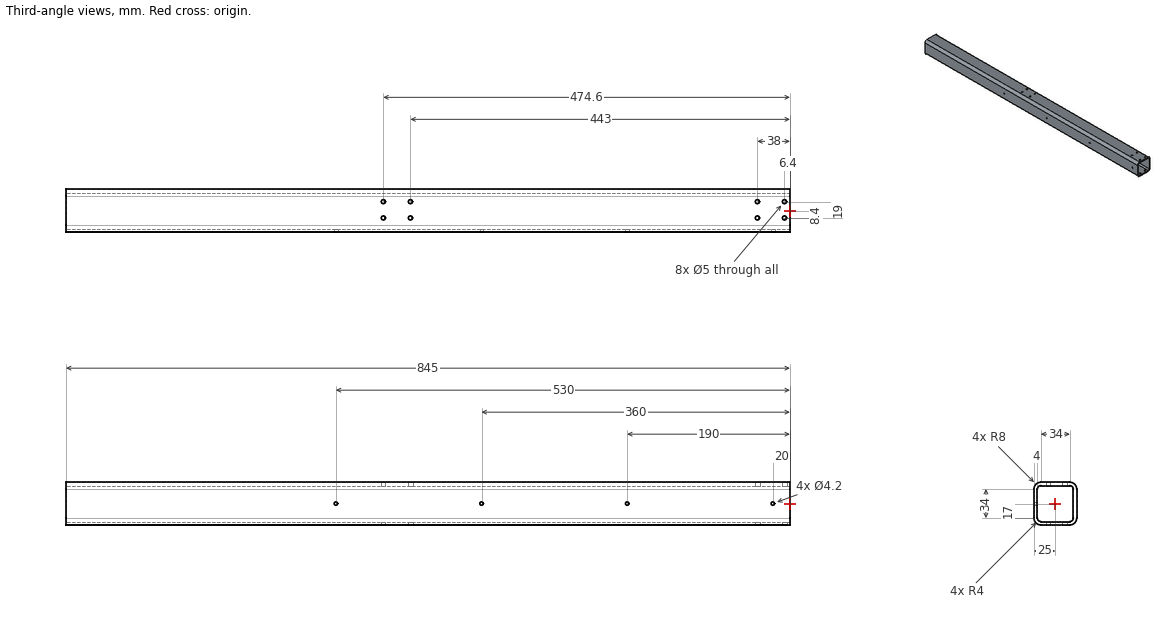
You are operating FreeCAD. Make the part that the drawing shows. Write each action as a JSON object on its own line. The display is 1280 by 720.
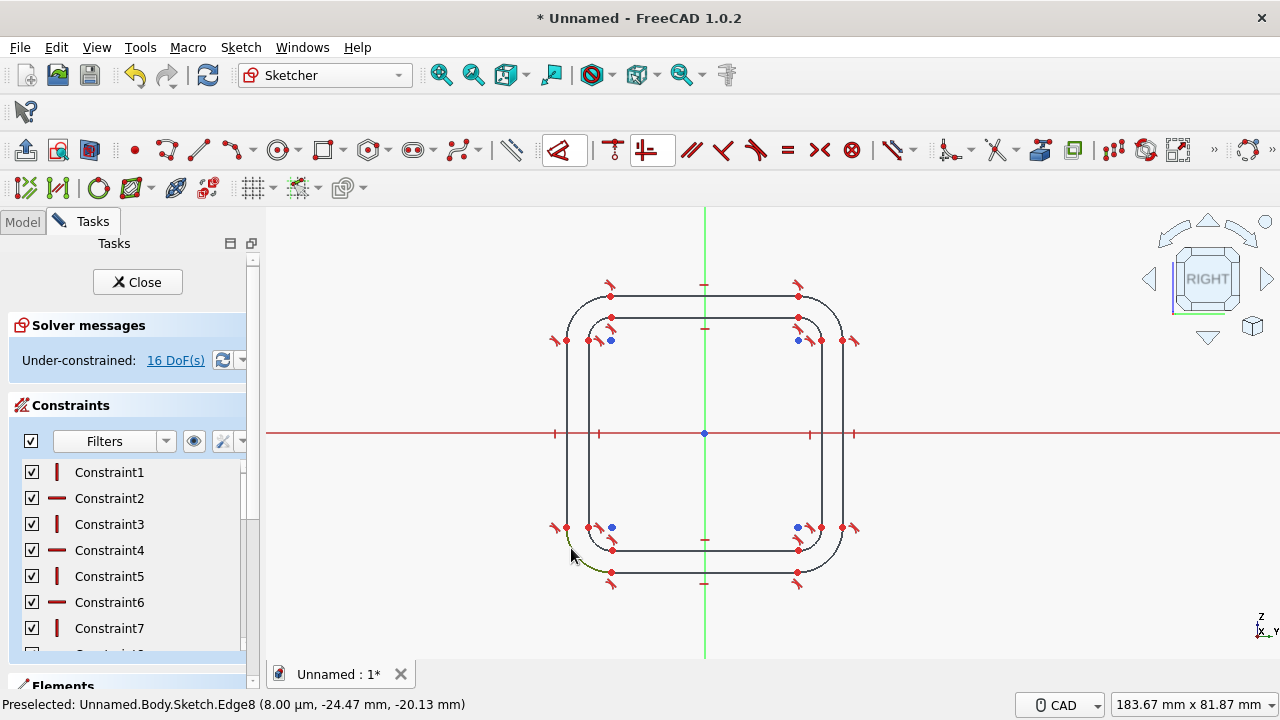
{"action": "scroll", "coordinate": [591, 538], "scroll_direction": "up", "scroll_amount": 2}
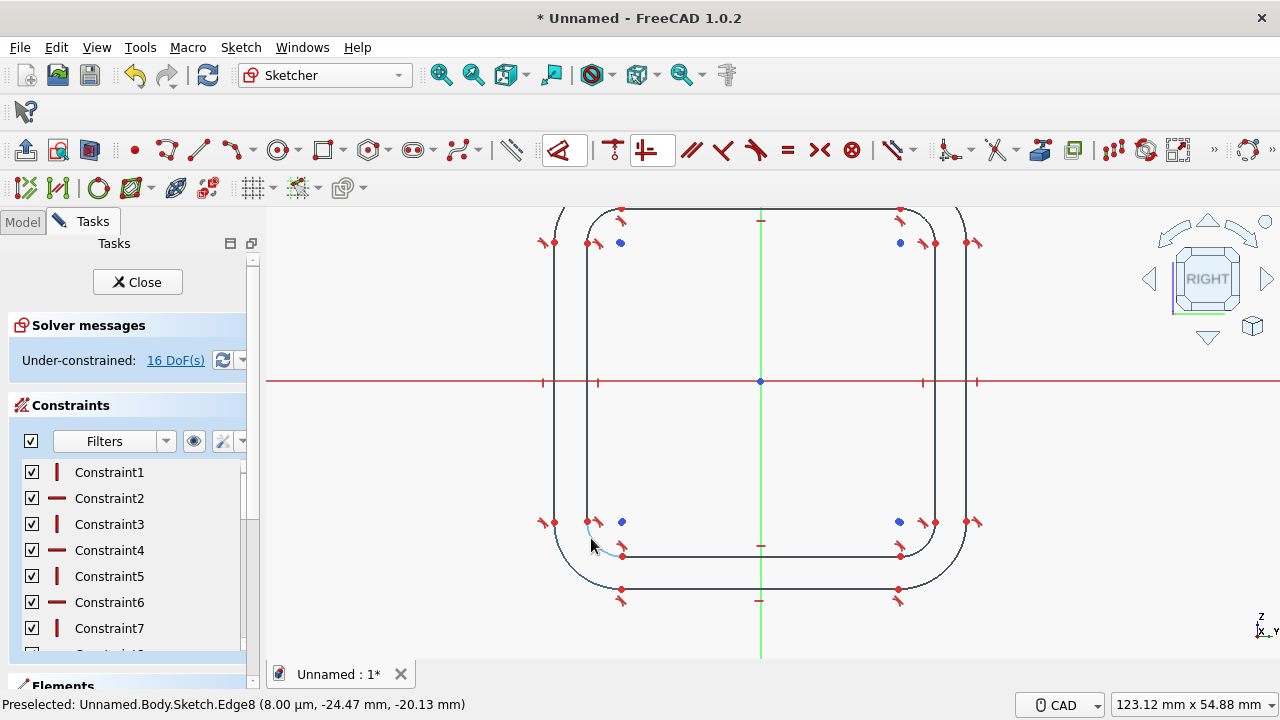
{"action": "left_click", "coordinate": [591, 537]}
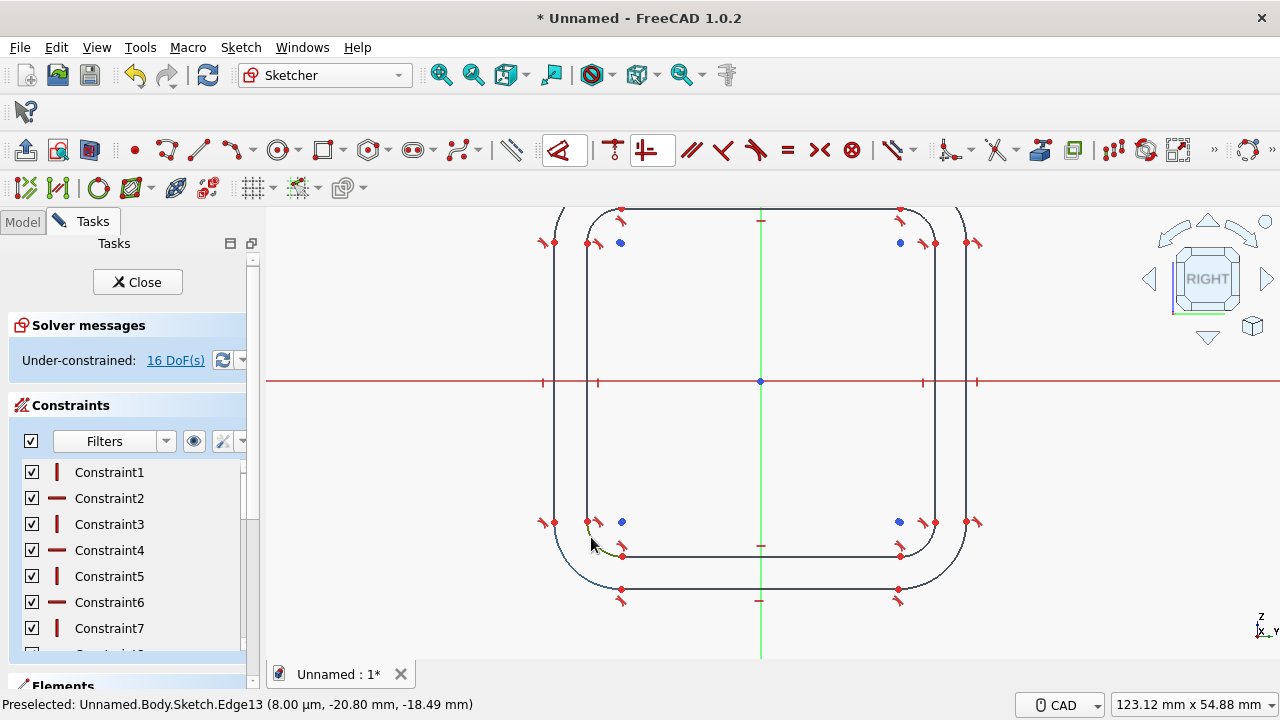
{"action": "left_click", "coordinate": [614, 150]}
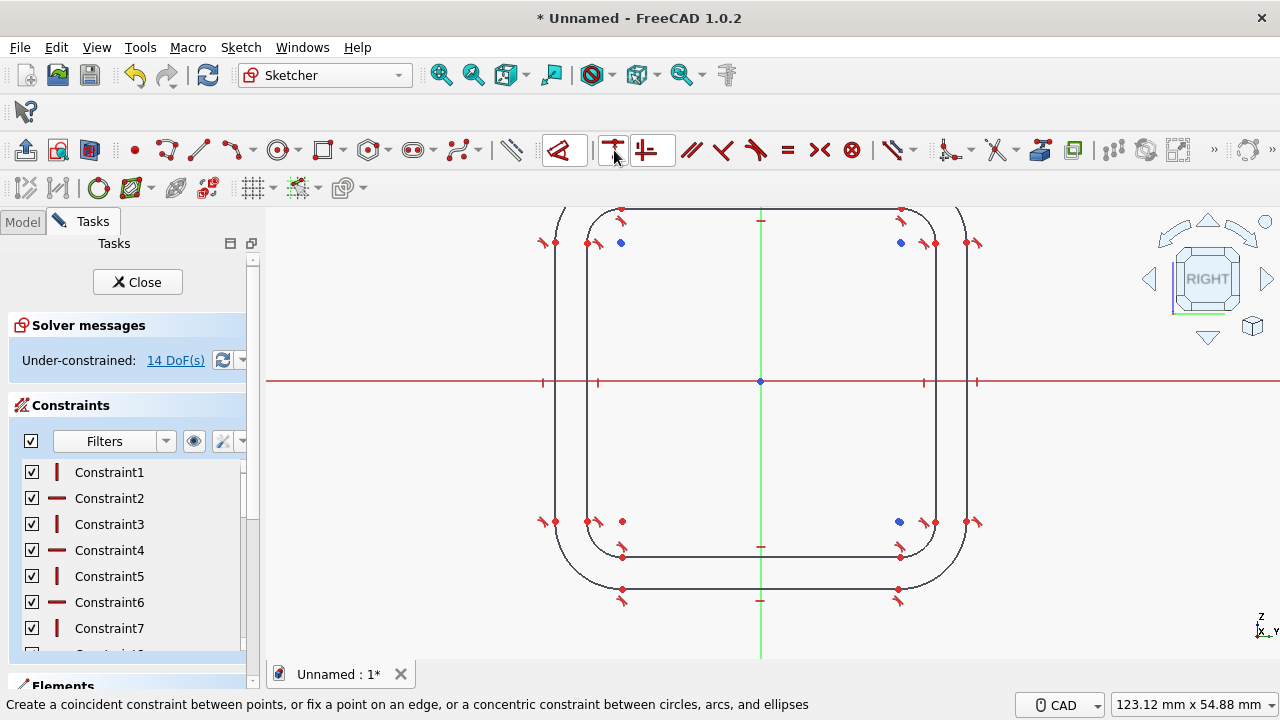
{"action": "left_click", "coordinate": [929, 582]}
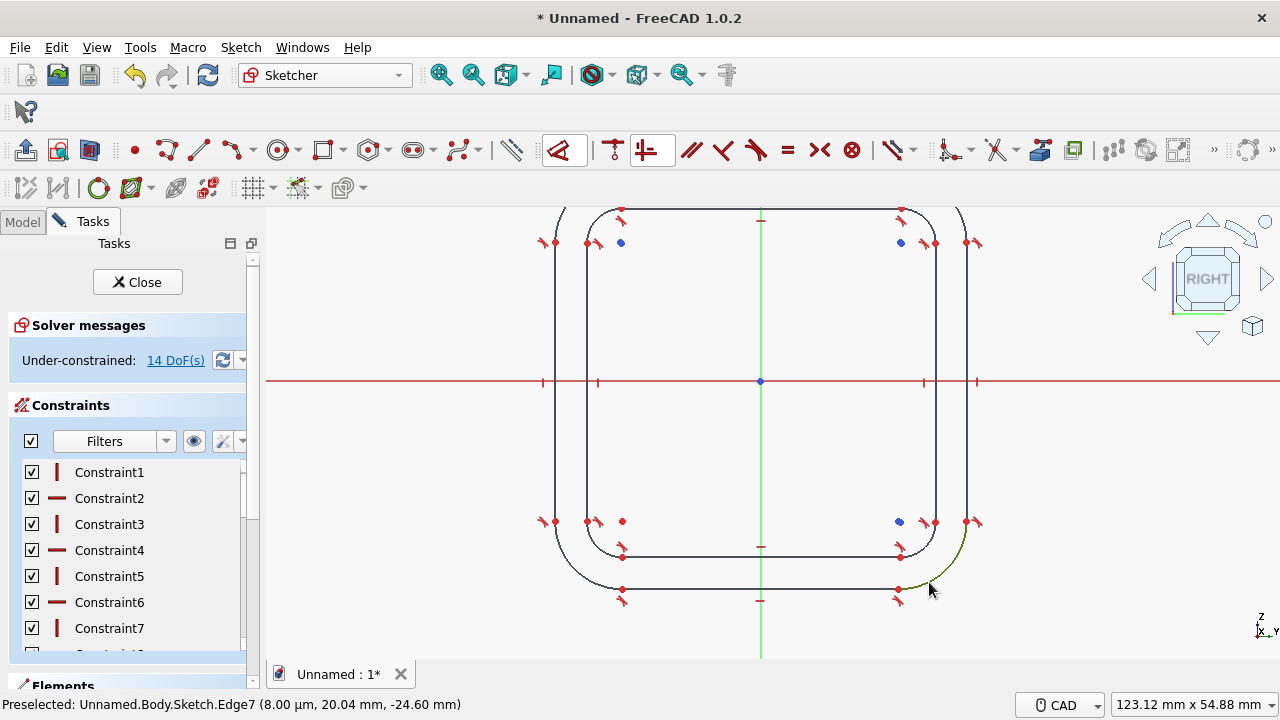
{"action": "left_click", "coordinate": [916, 554]}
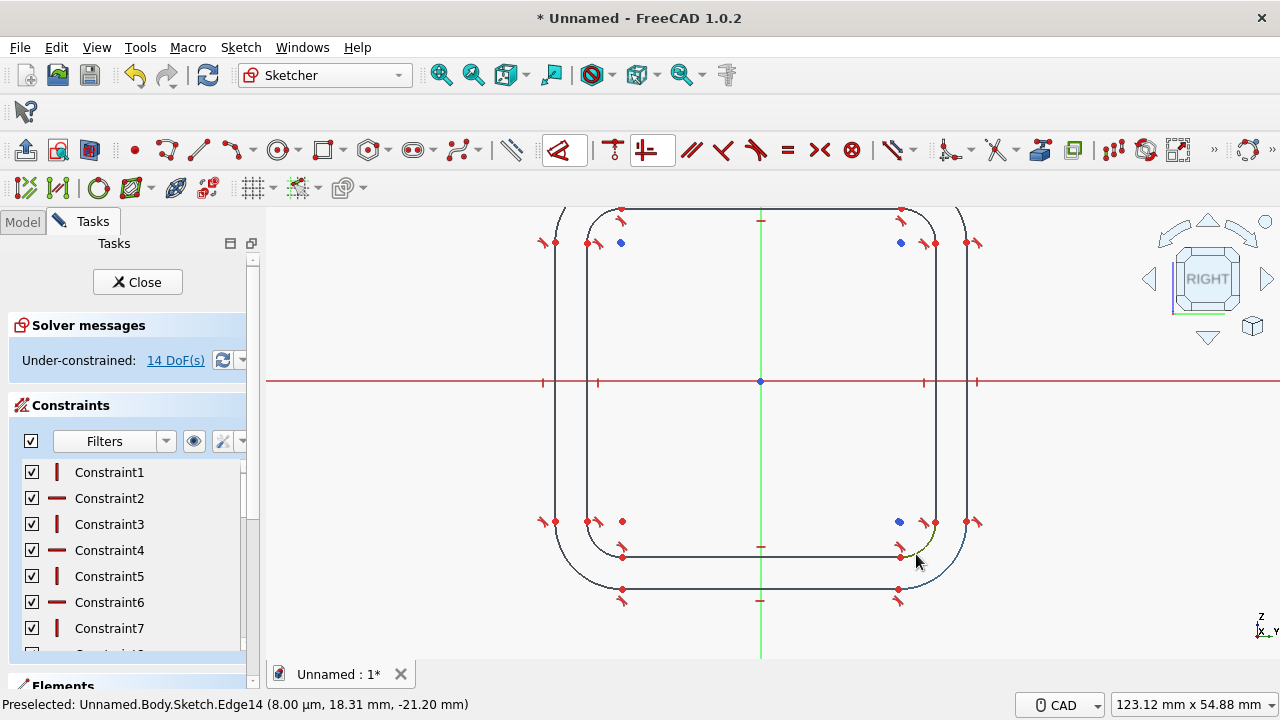
{"action": "left_click", "coordinate": [614, 150]}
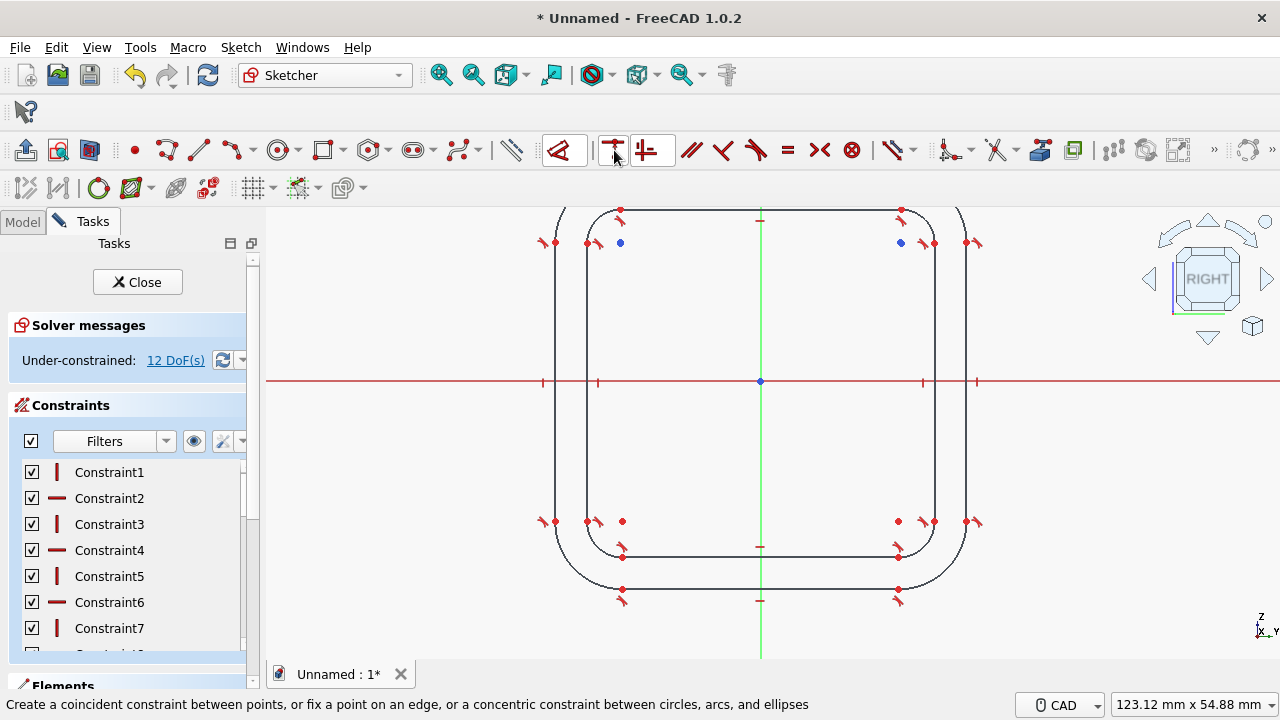
{"action": "scroll", "coordinate": [591, 539], "scroll_direction": "down", "scroll_amount": 2}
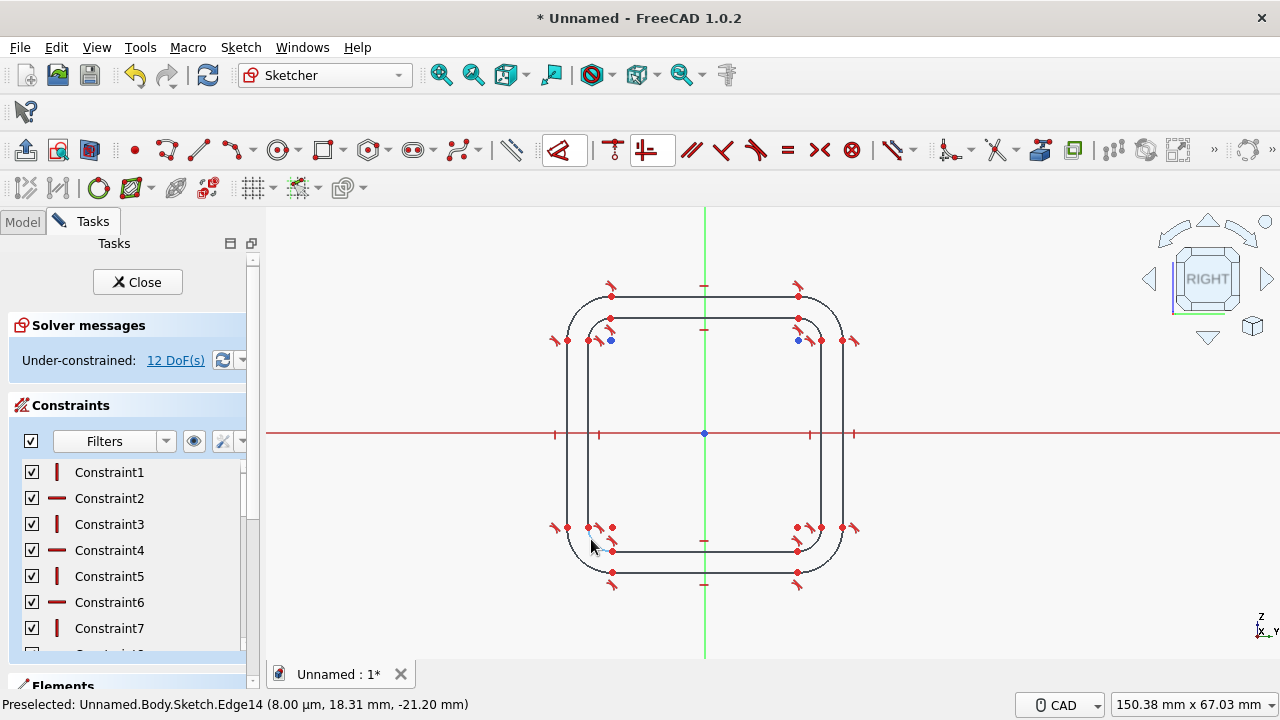
{"action": "left_click", "coordinate": [838, 321]}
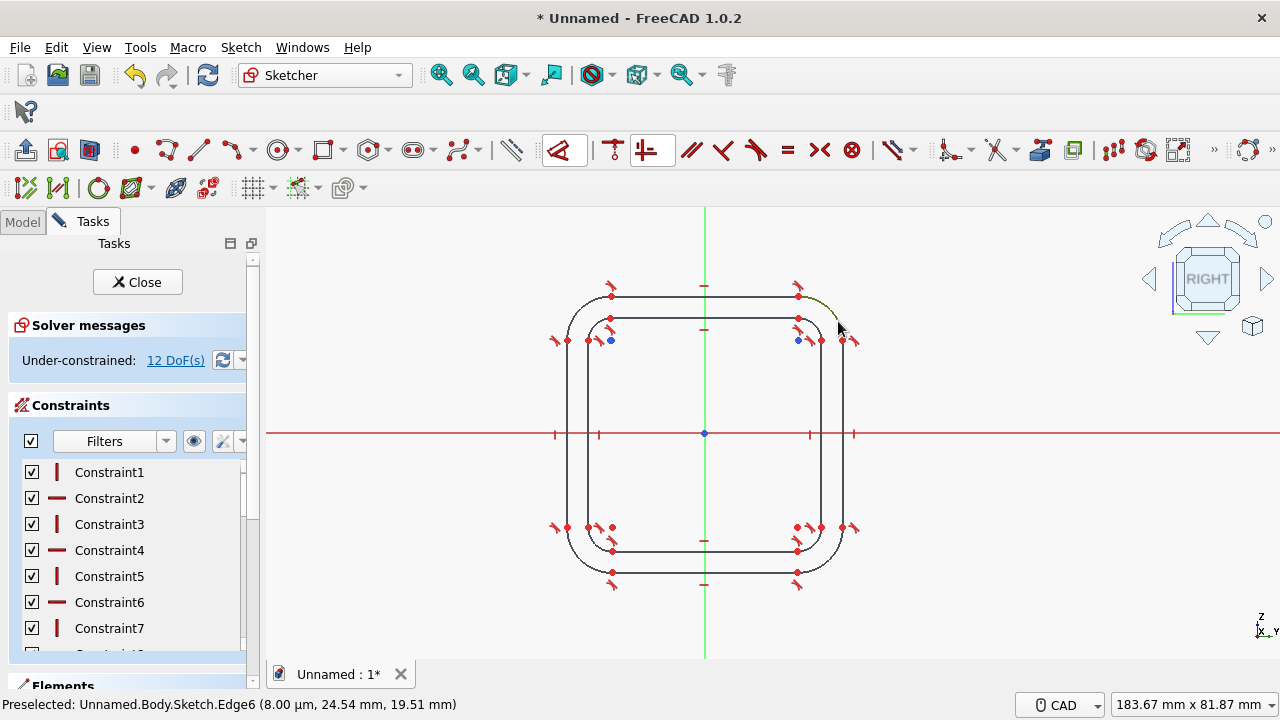
{"action": "scroll", "coordinate": [819, 331], "scroll_direction": "up", "scroll_amount": 2}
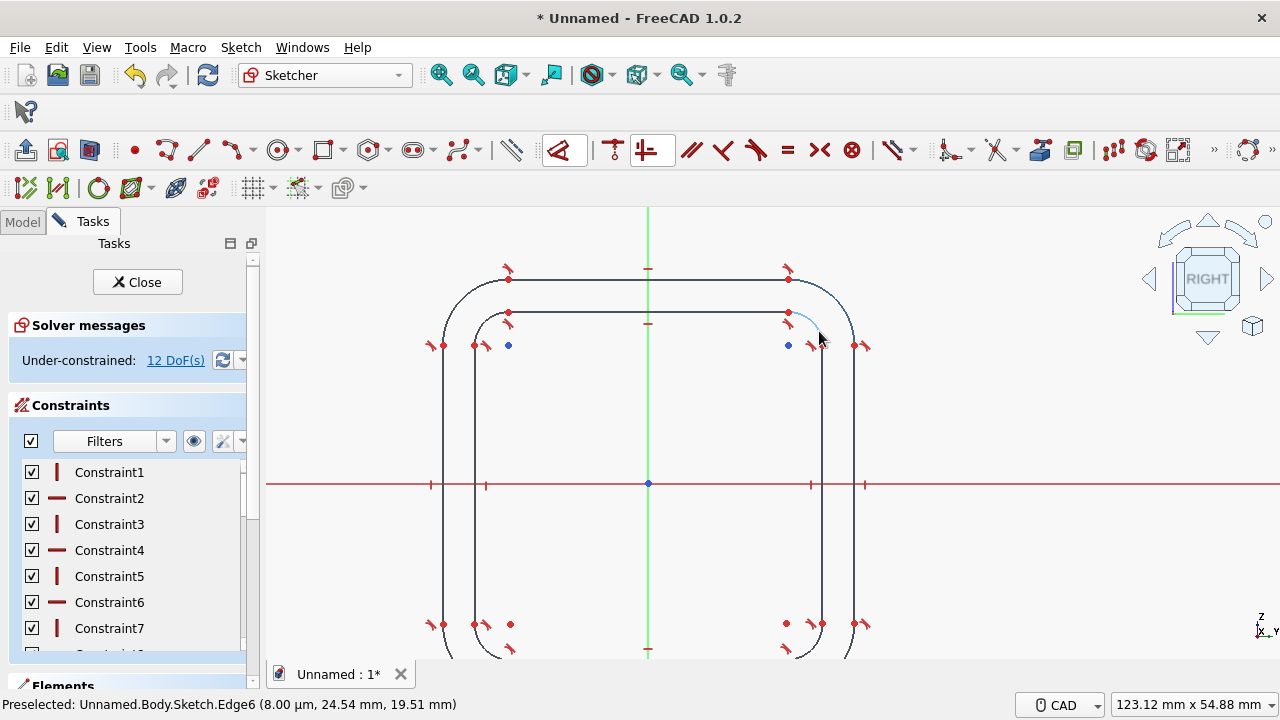
{"action": "left_click", "coordinate": [819, 331]}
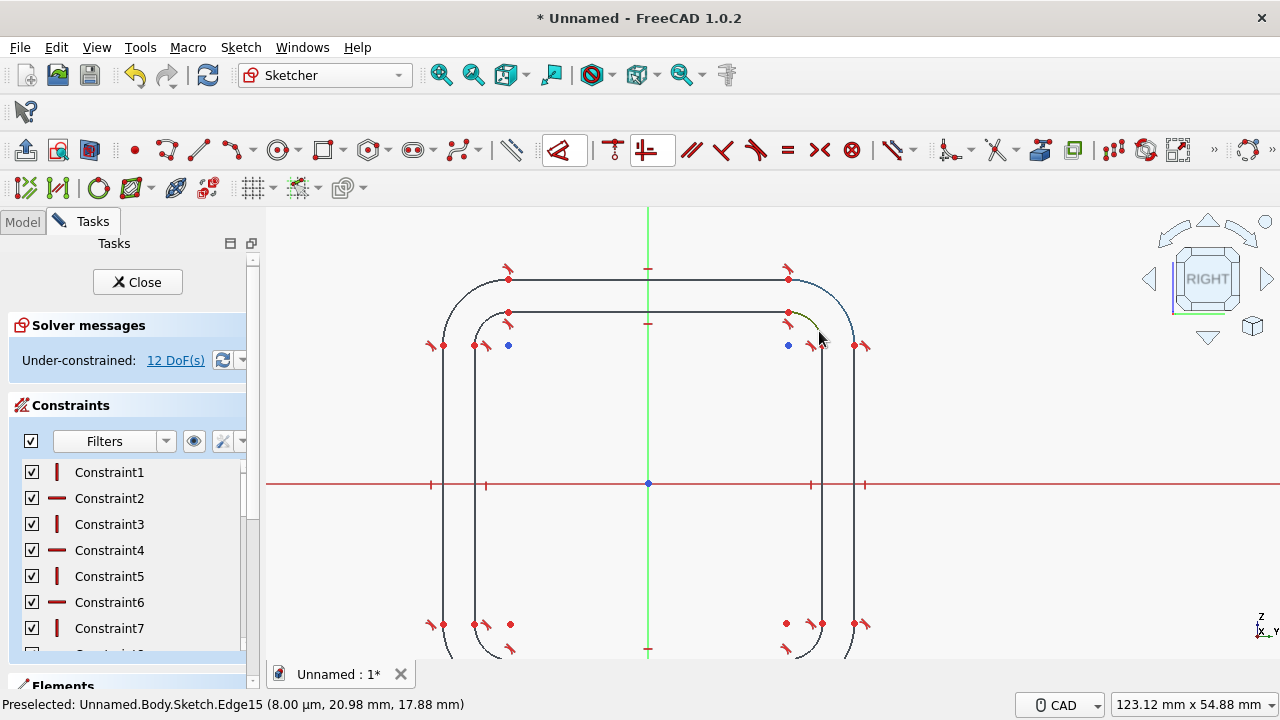
{"action": "left_click", "coordinate": [614, 150]}